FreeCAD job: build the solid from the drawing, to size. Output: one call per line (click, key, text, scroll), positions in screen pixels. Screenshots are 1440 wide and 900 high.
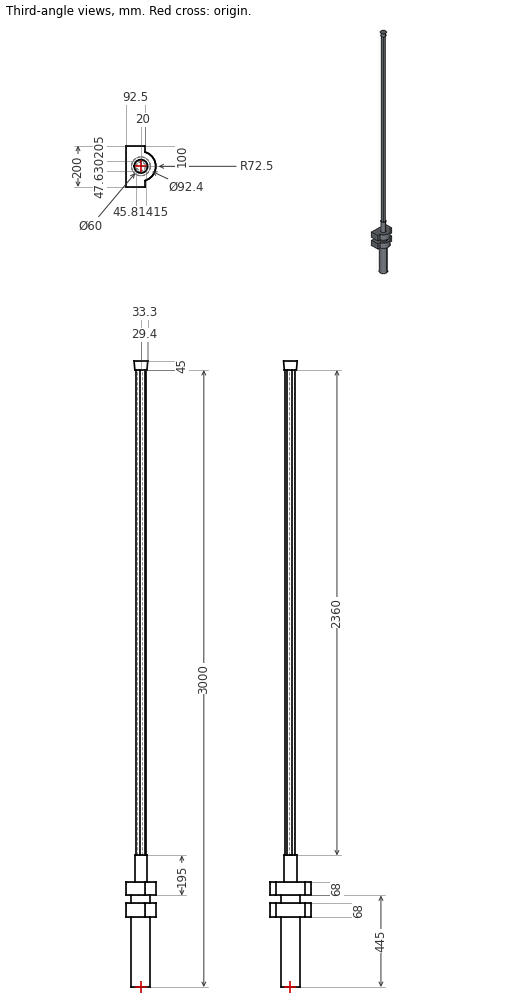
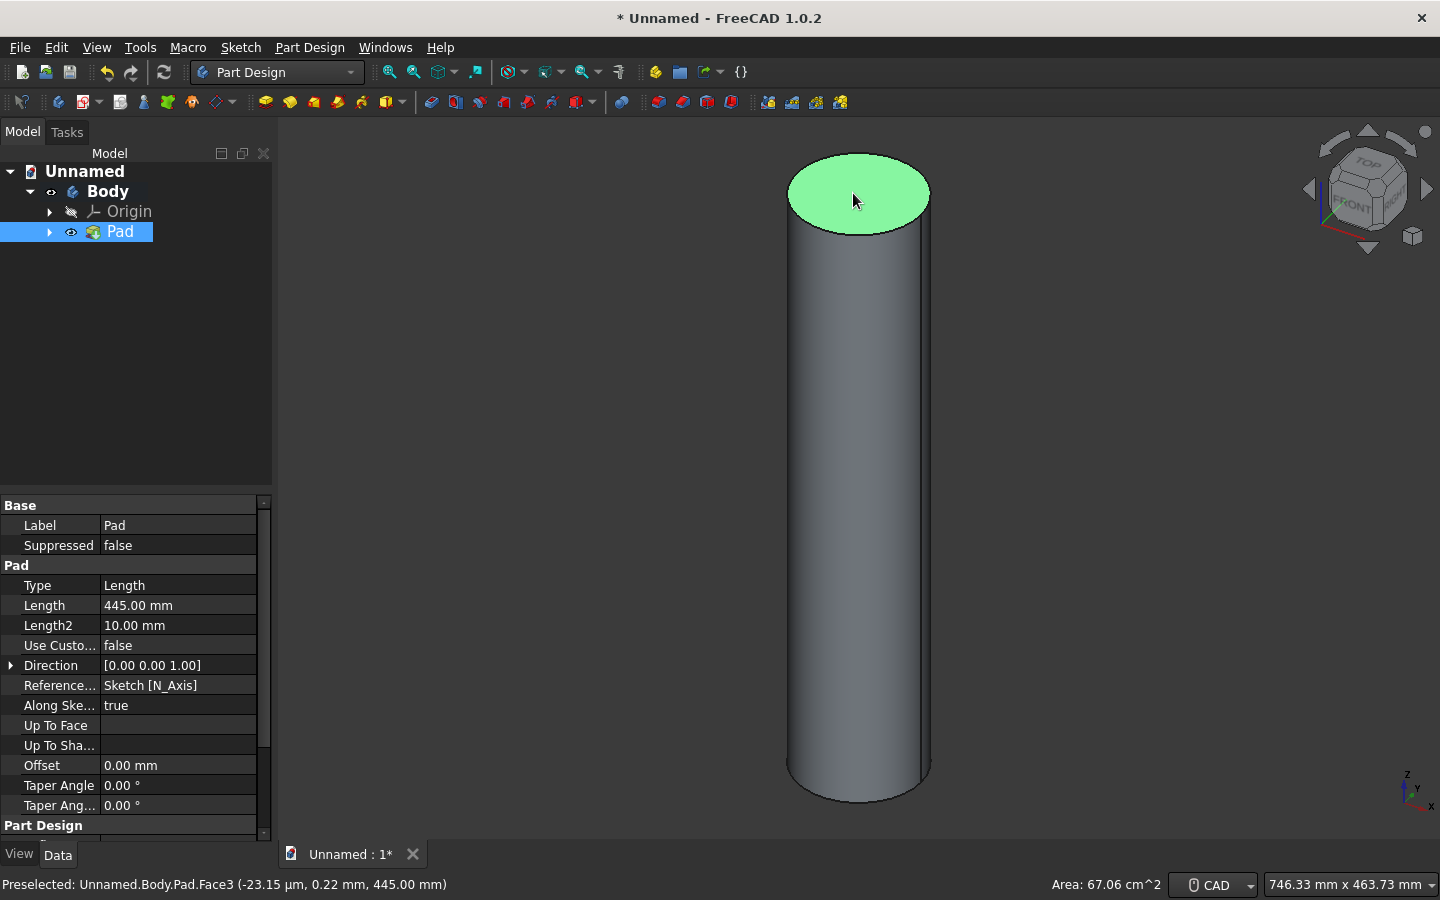
click(84, 102)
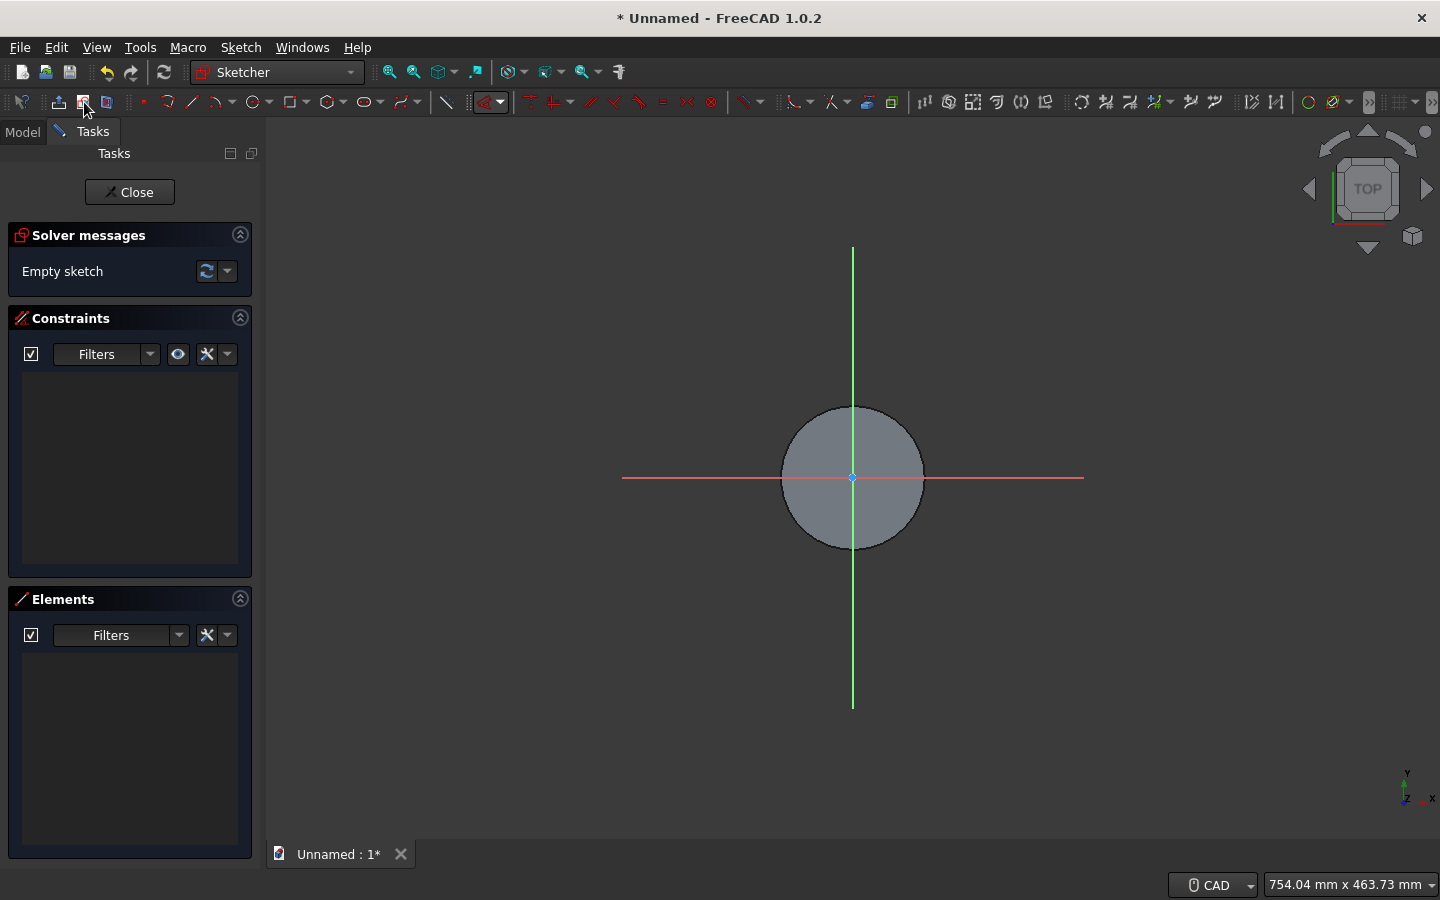
scroll(870, 478, up, 8)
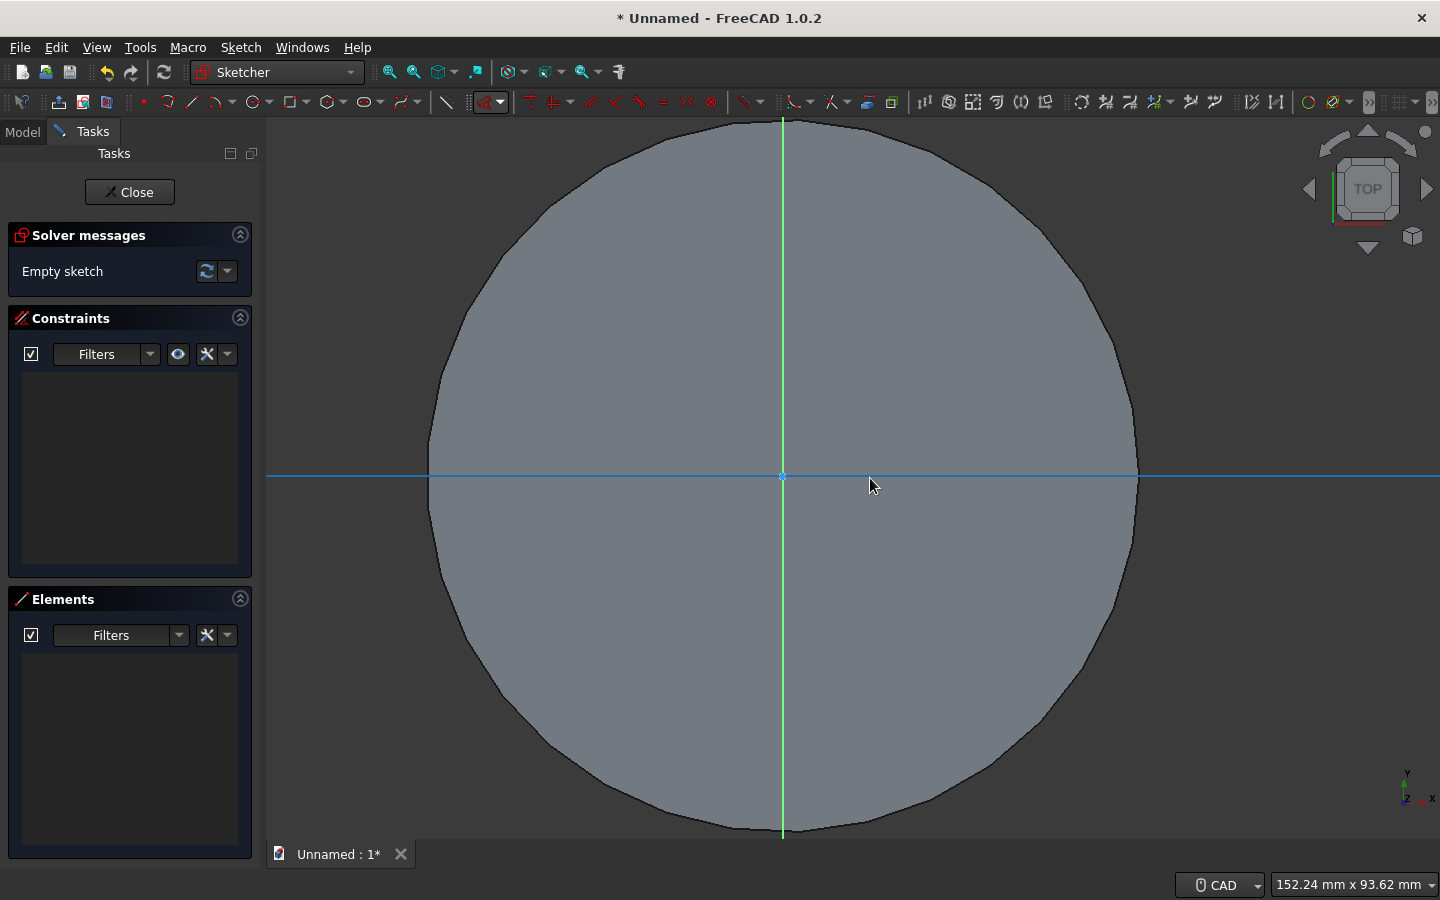
key(g)
key(c)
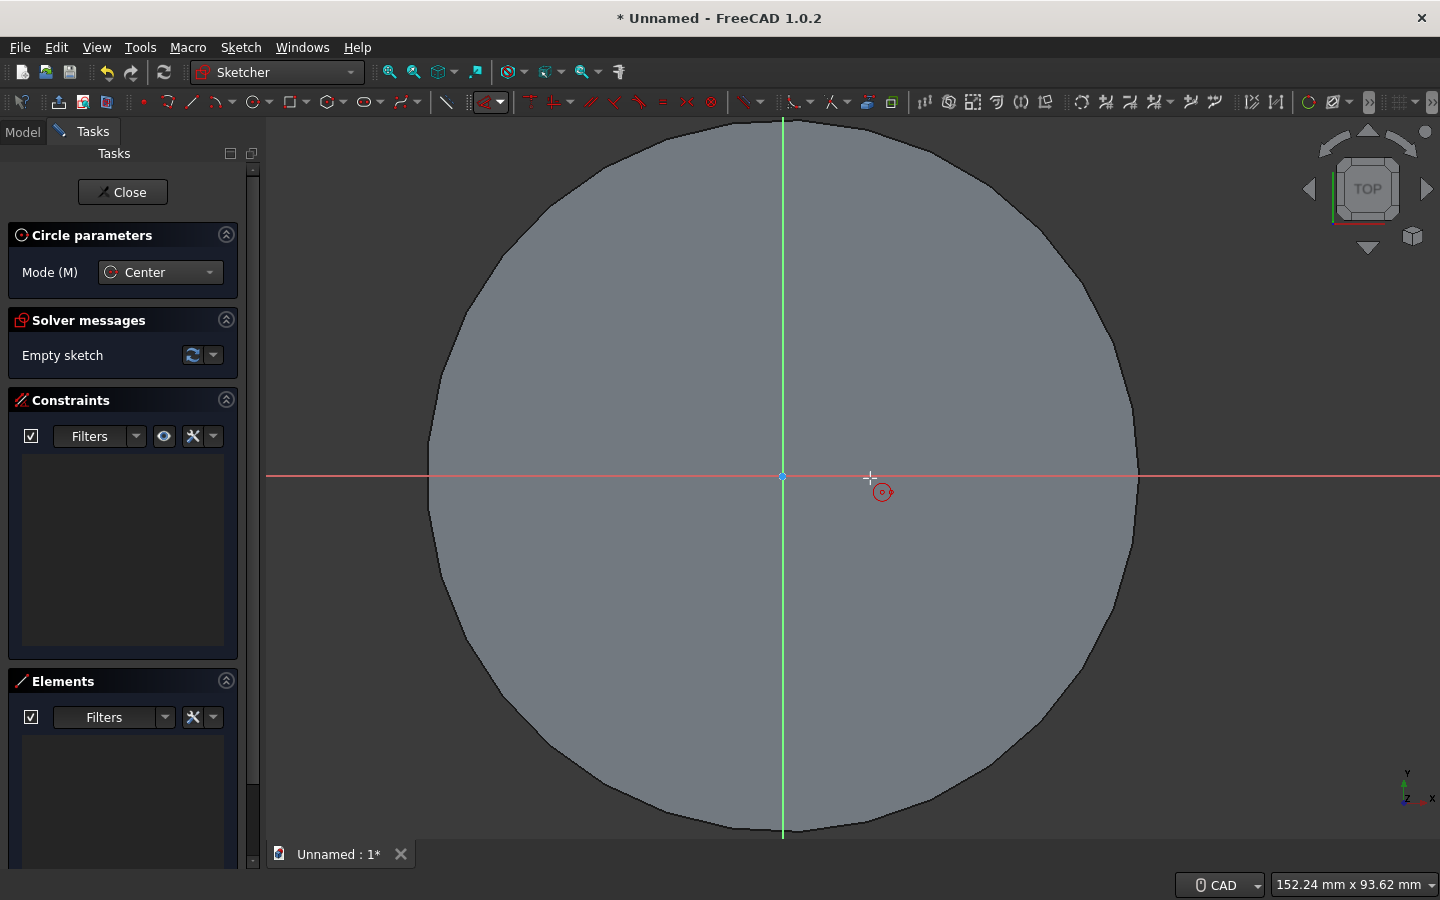
click(783, 476)
click(947, 312)
key(Escape)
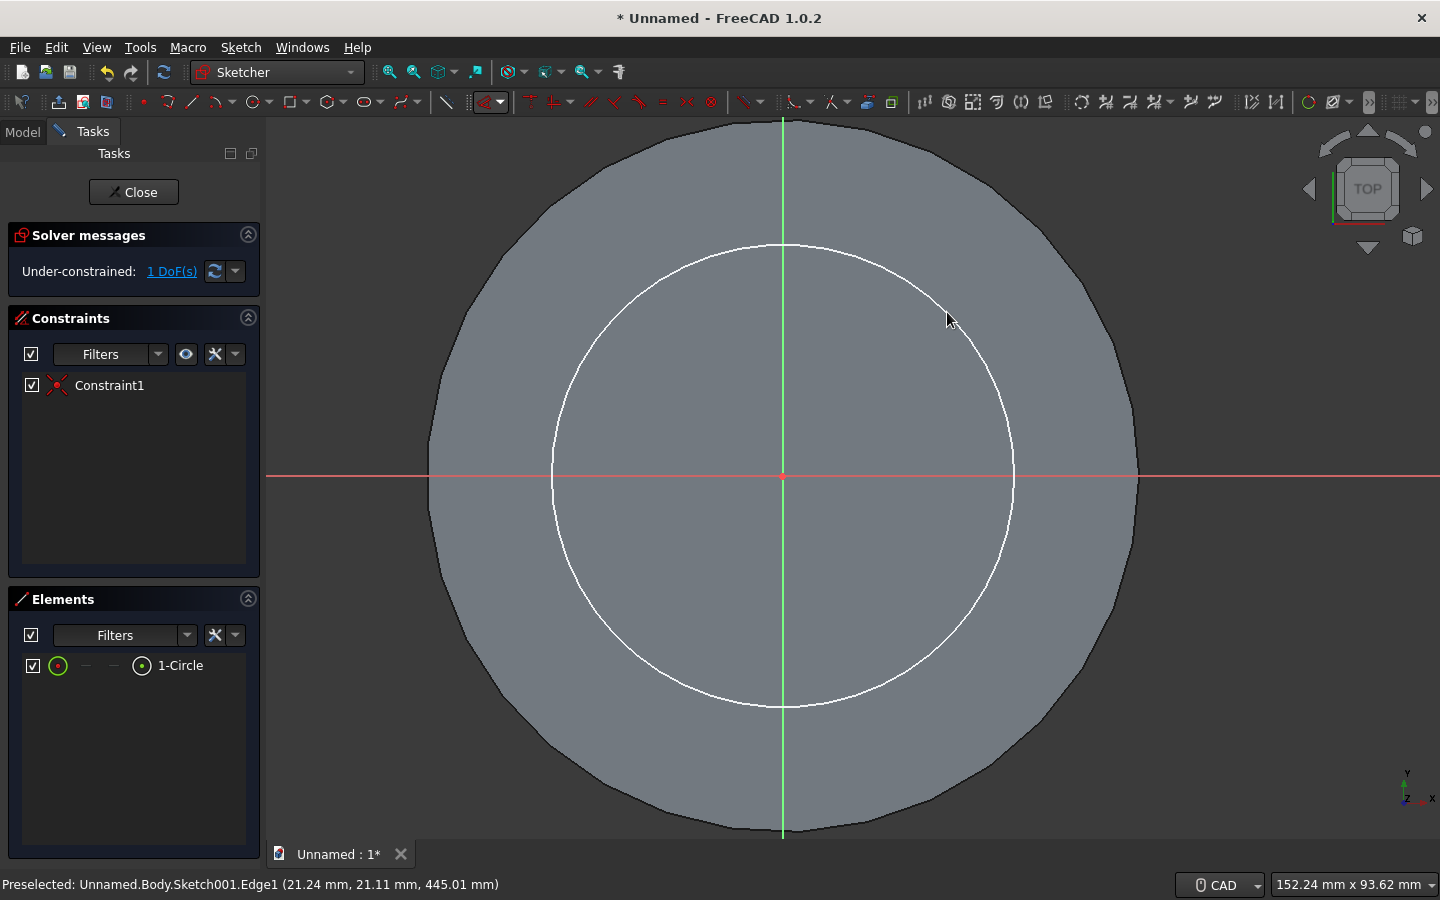
click(946, 312)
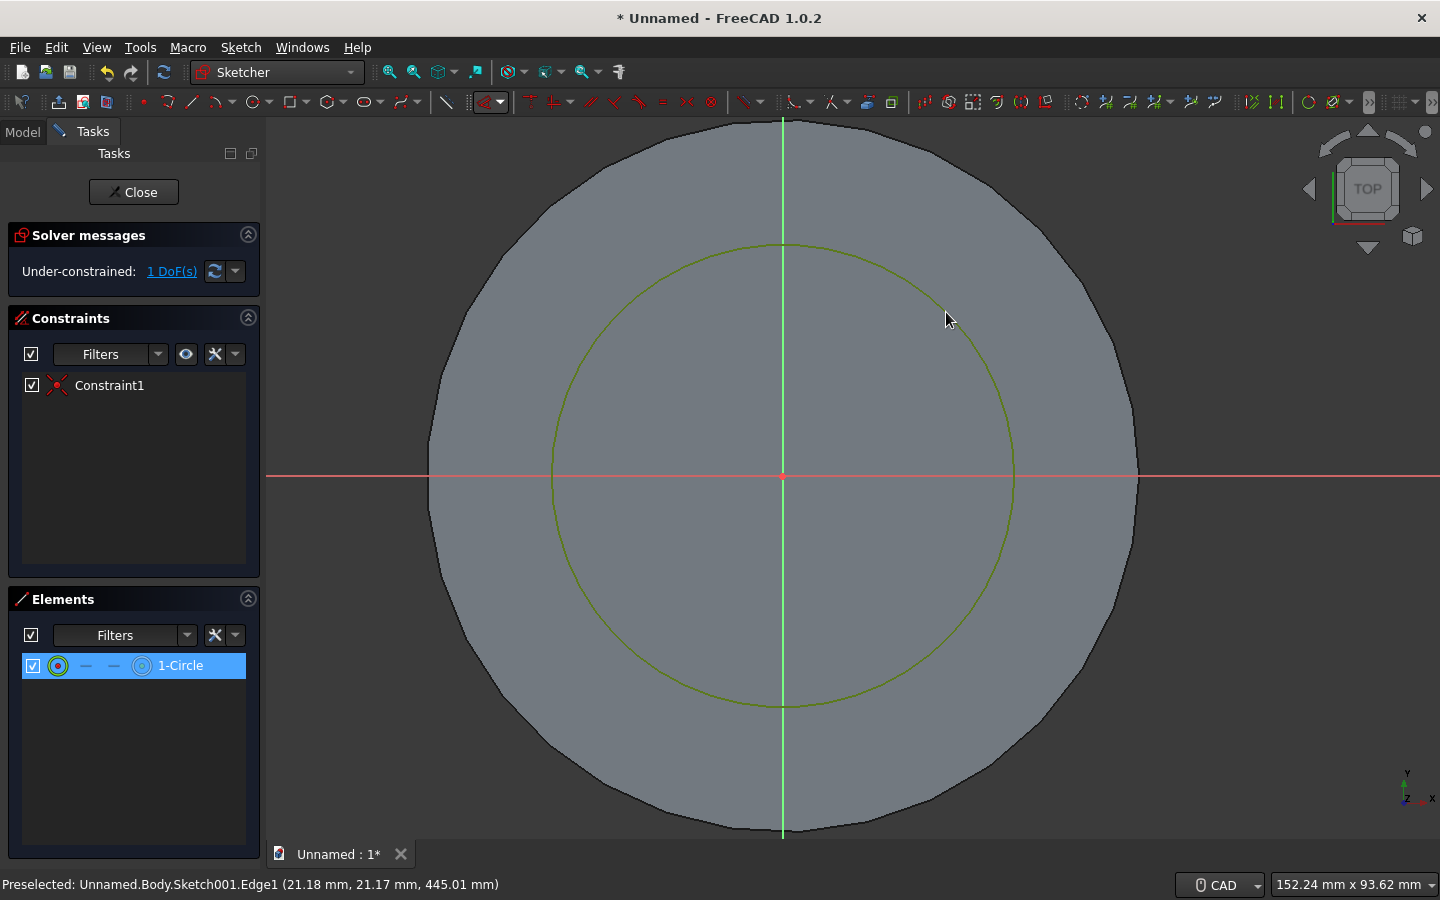
key(k)
key(o)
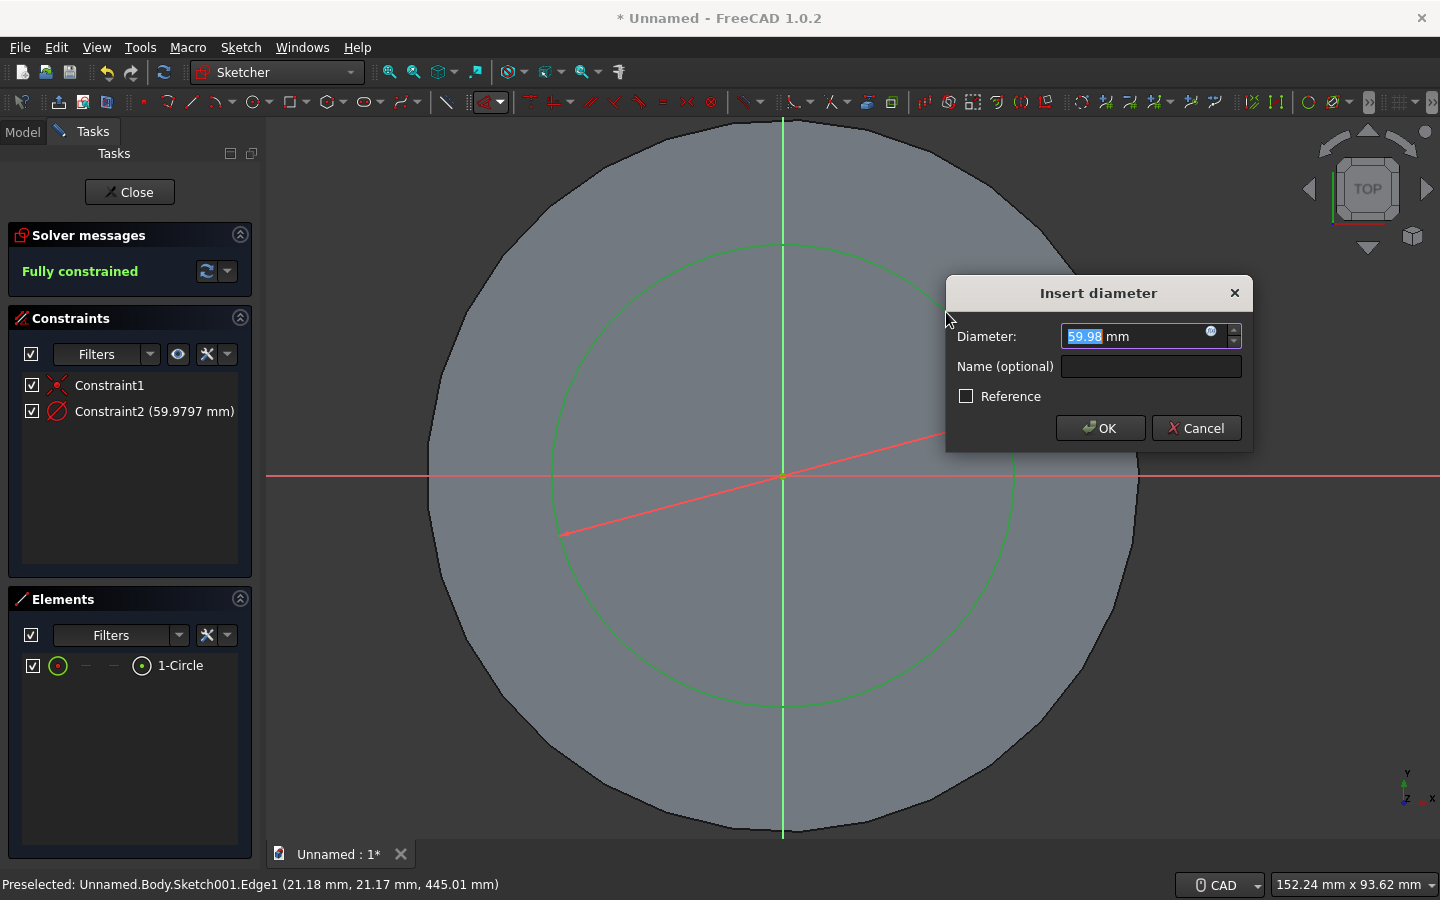
text(60)
key(Return)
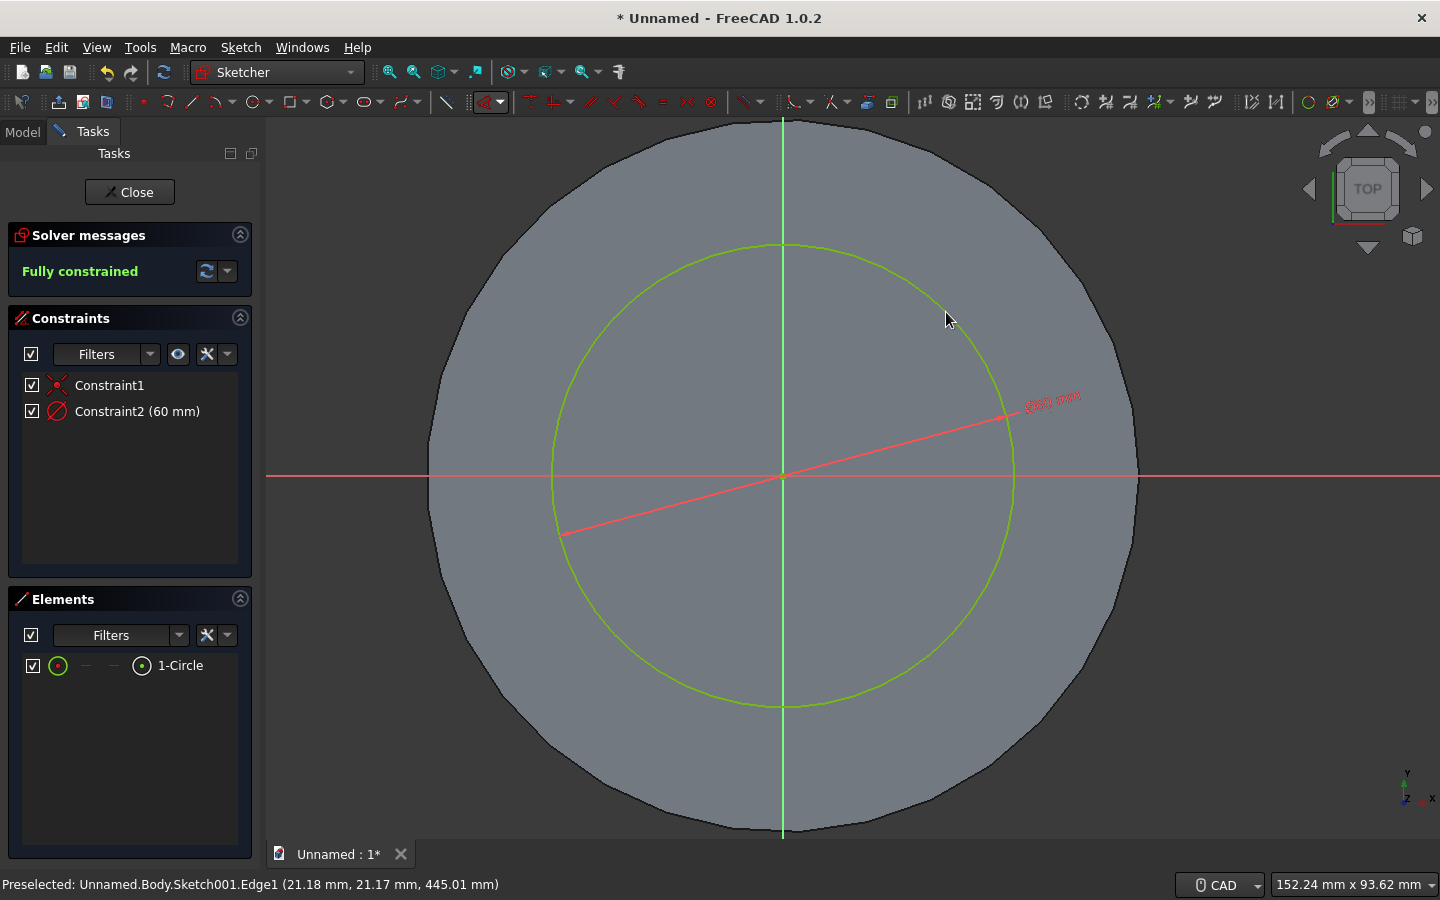
click(130, 192)